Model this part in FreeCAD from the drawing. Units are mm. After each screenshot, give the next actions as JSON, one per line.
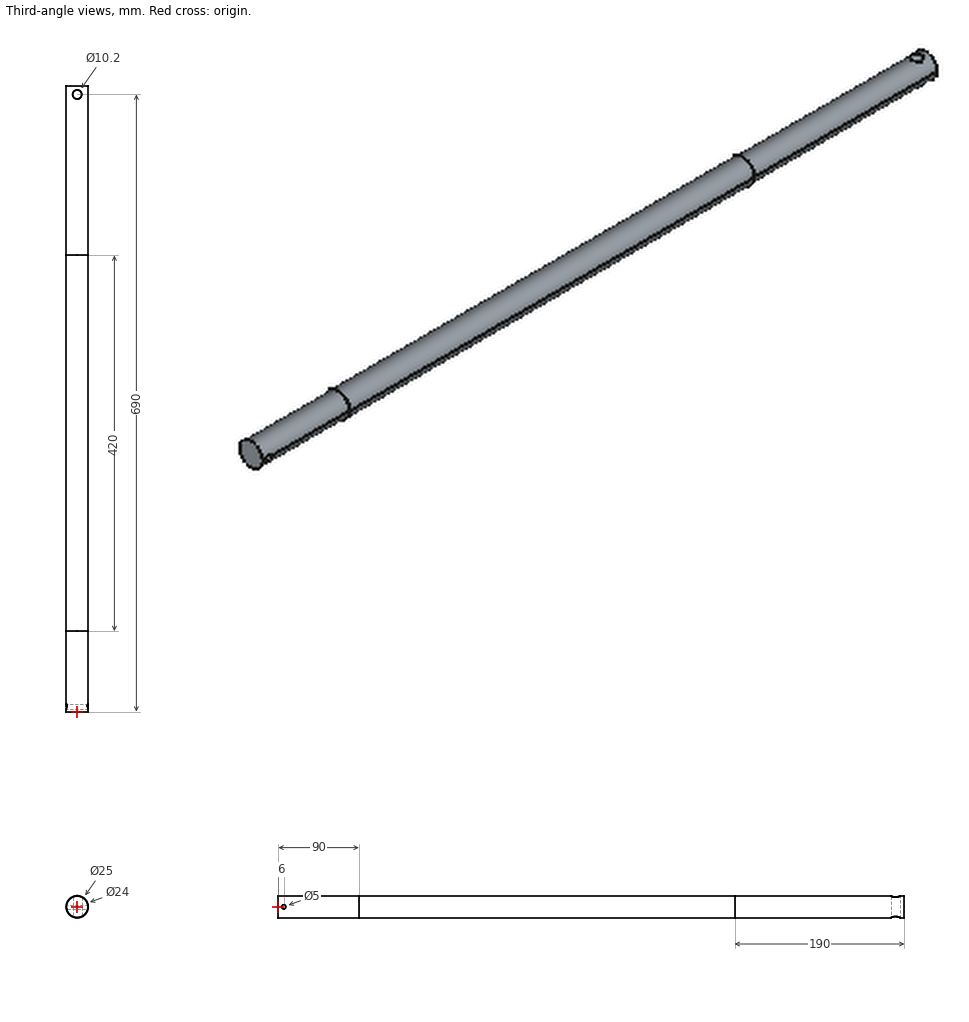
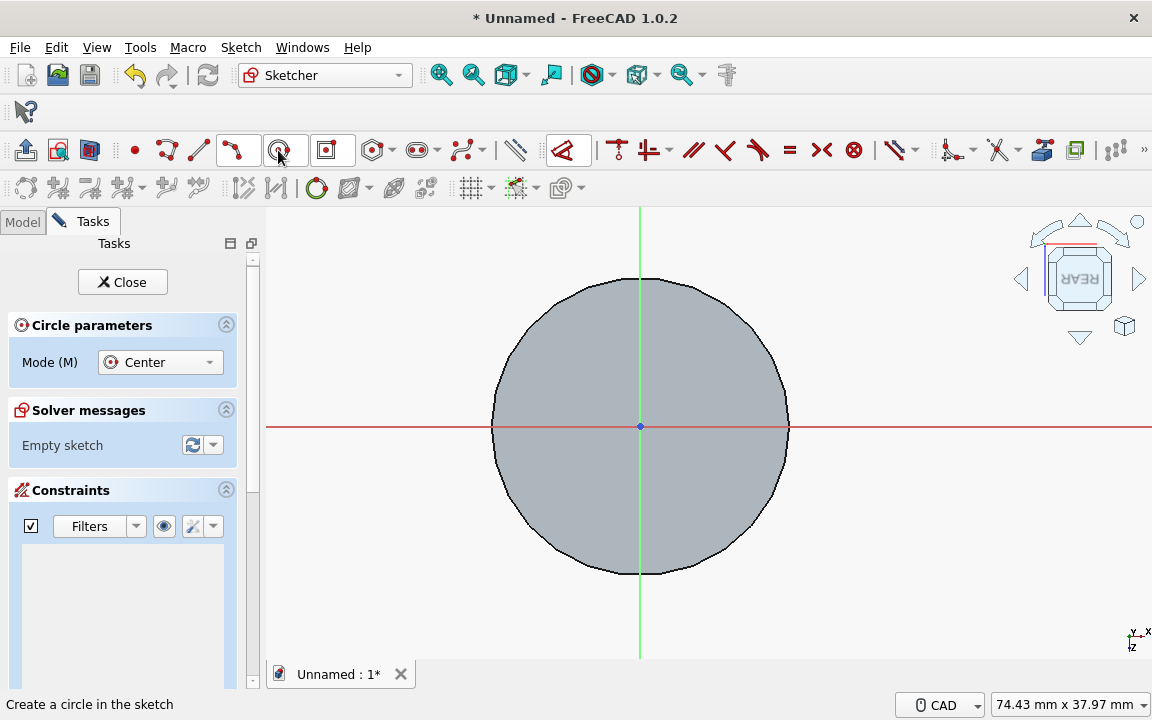
{"action": "left_click", "coordinate": [640, 427]}
{"action": "left_click", "coordinate": [741, 326]}
{"action": "key", "text": "Escape"}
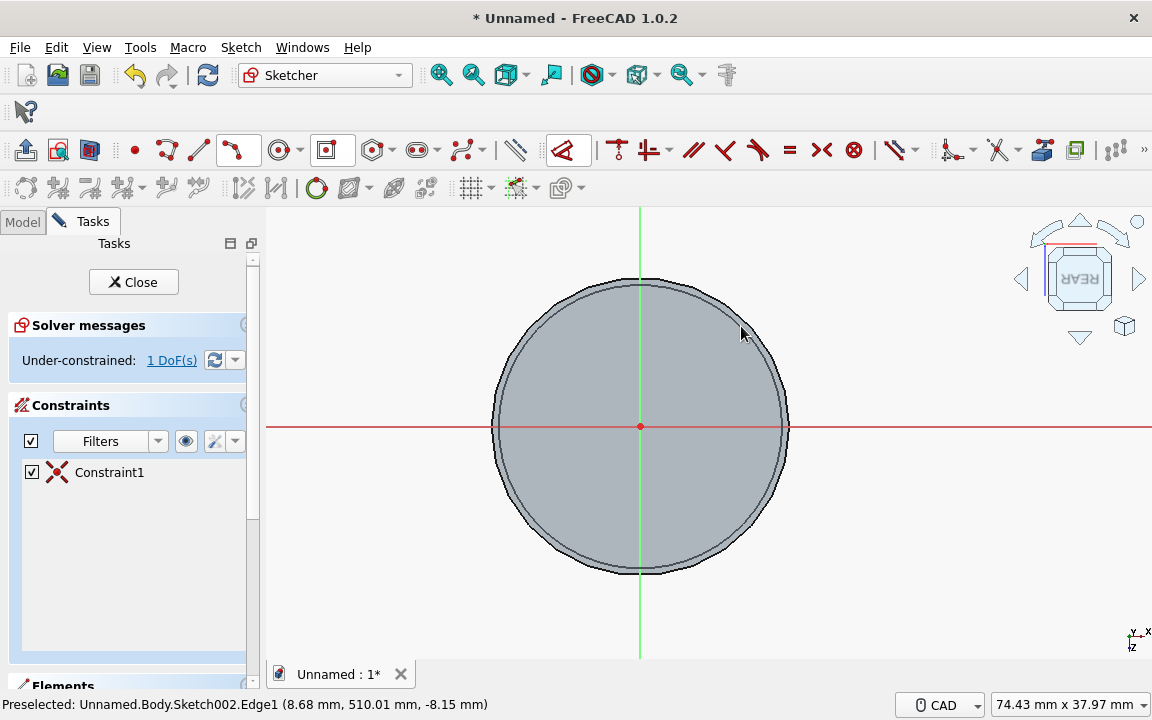
{"action": "left_click", "coordinate": [740, 326]}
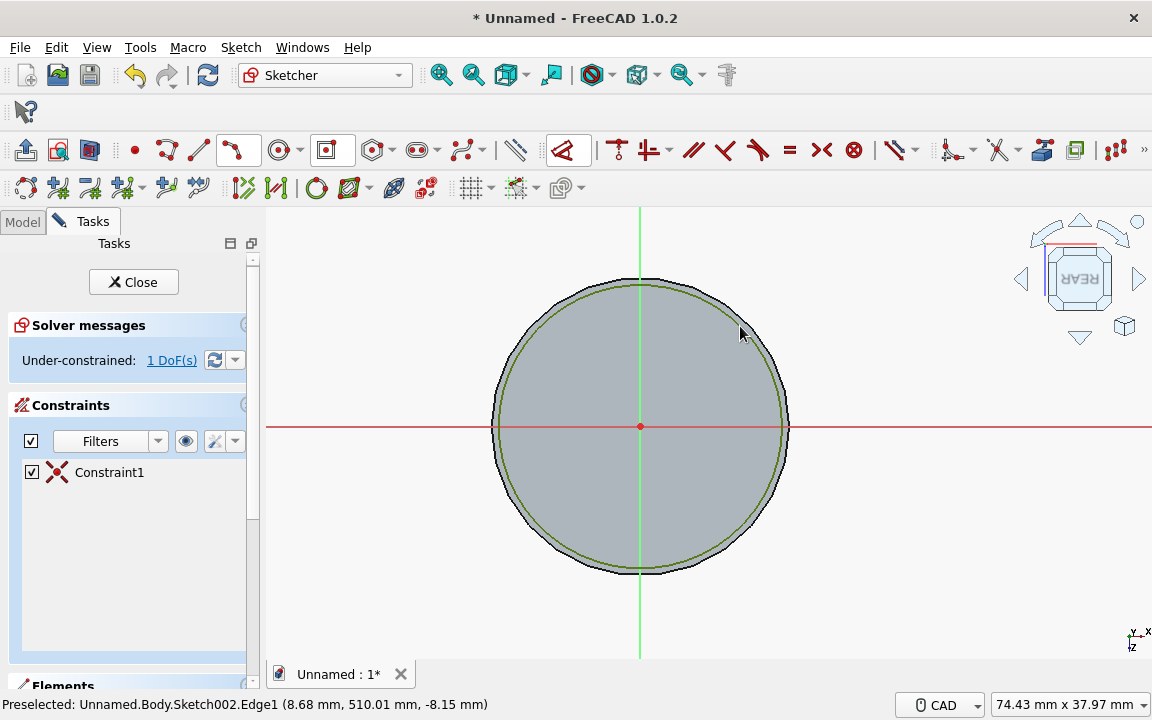
{"action": "key", "text": "k o"}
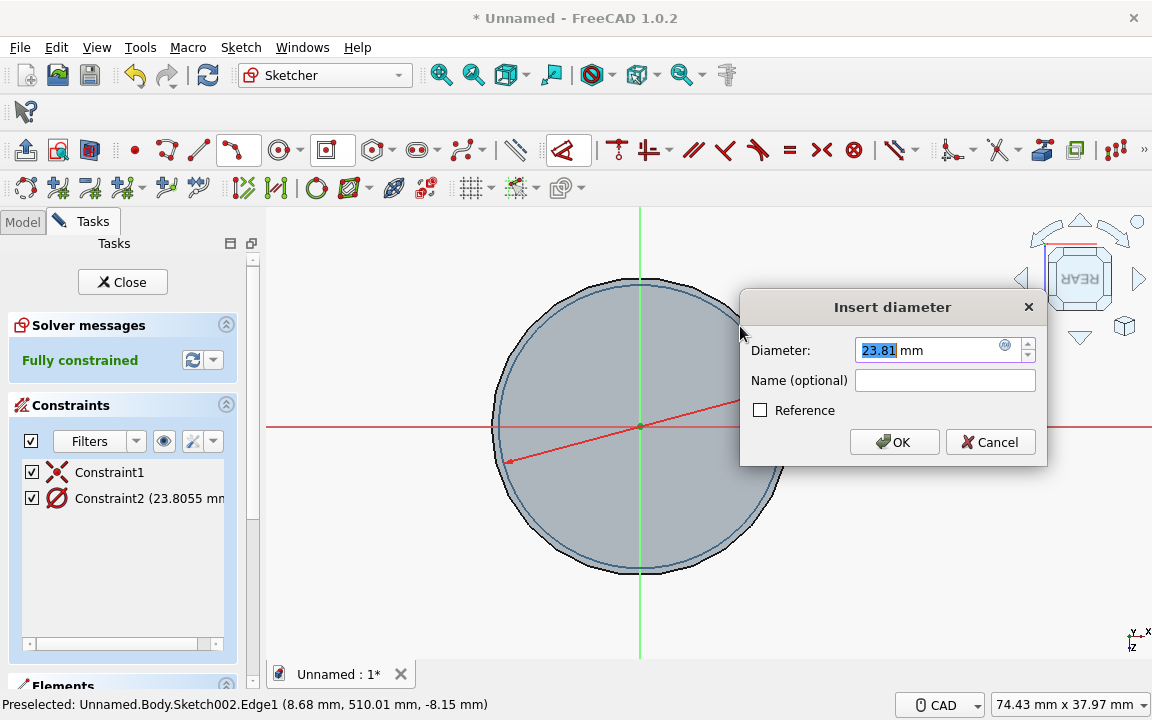
{"action": "type", "text": "24"}
{"action": "key", "text": "Return"}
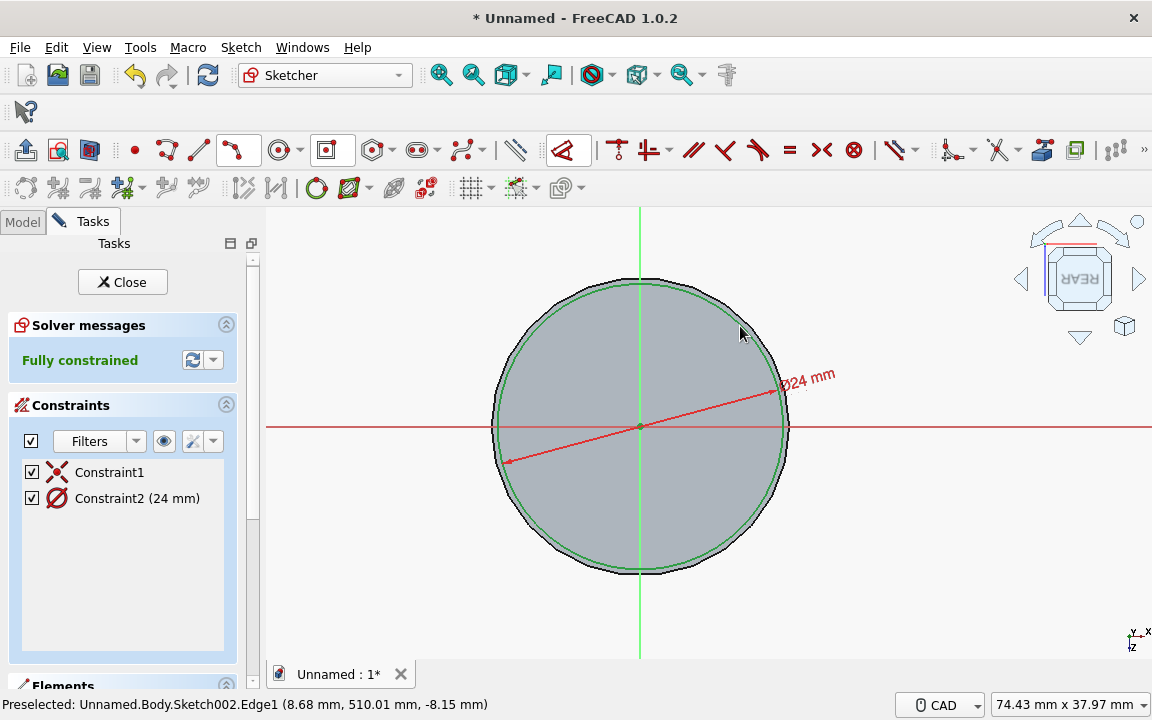
{"action": "left_click", "coordinate": [123, 282]}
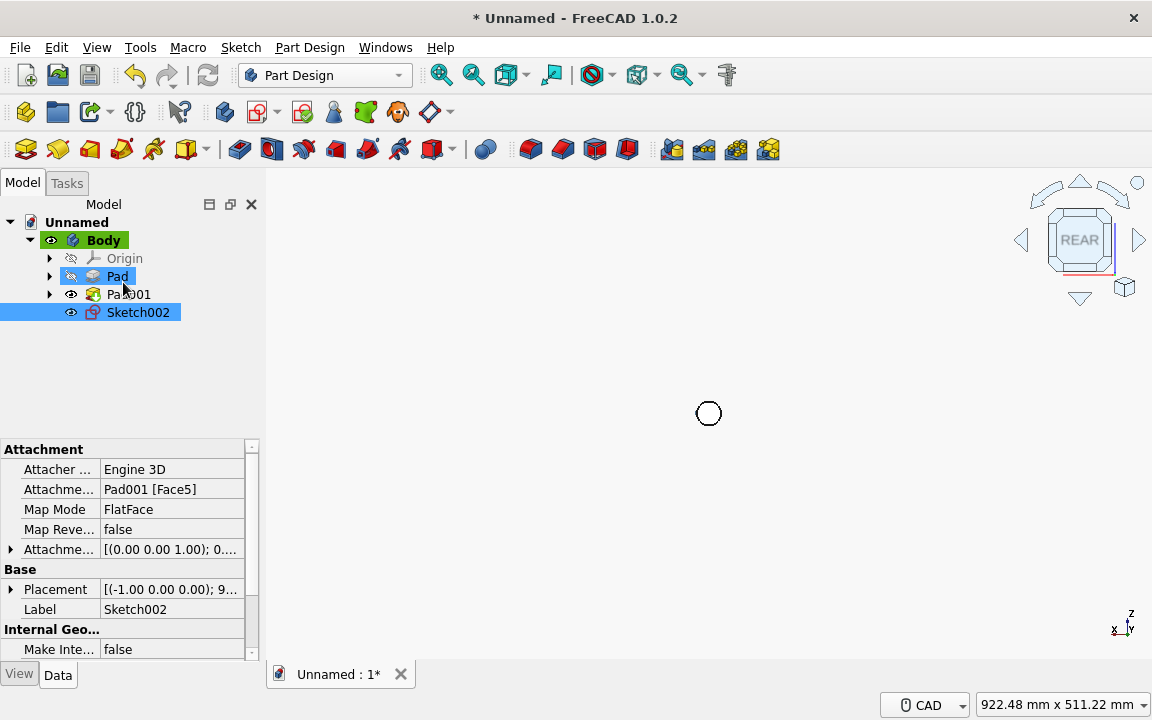
{"action": "left_click", "coordinate": [26, 150]}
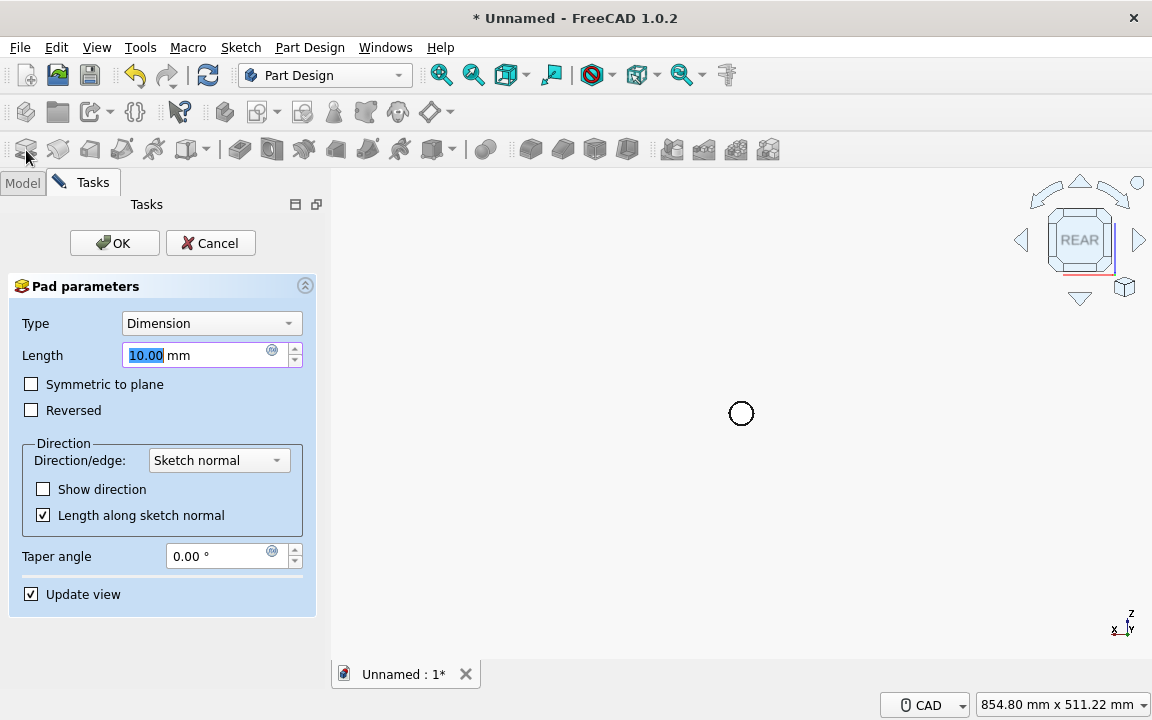
{"action": "type", "text": "190"}
{"action": "key", "text": "Tab"}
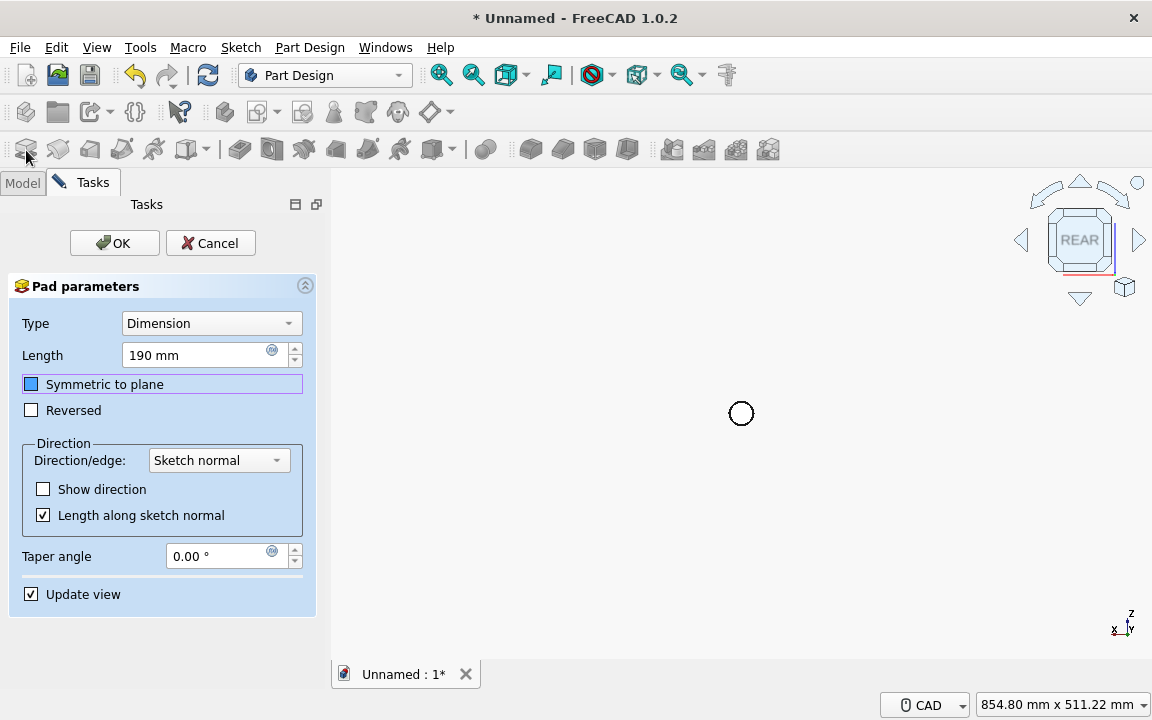
{"action": "left_click", "coordinate": [115, 243]}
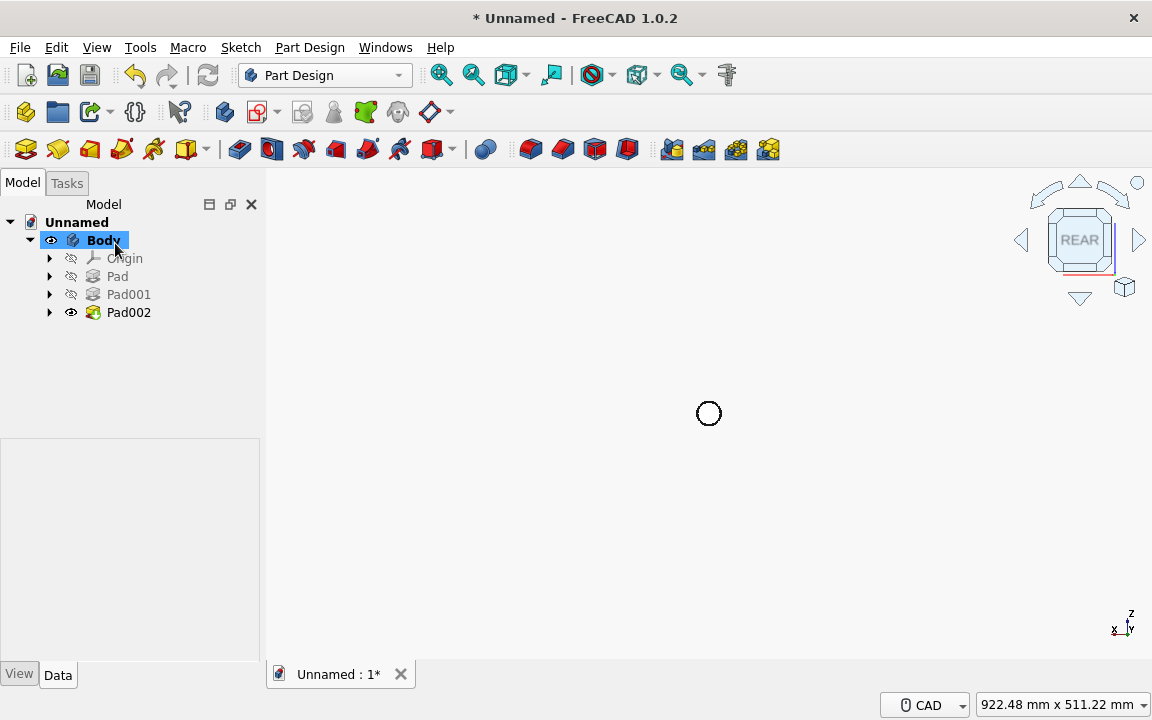
{"action": "left_click", "coordinate": [442, 76]}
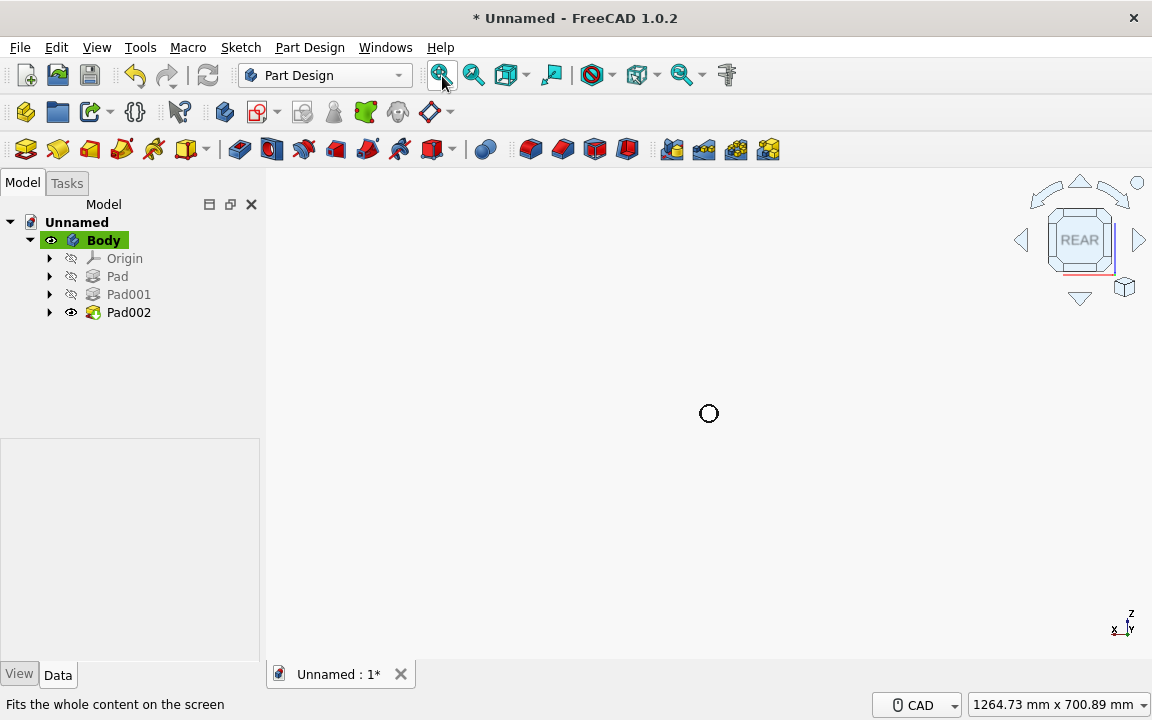
{"action": "left_click", "coordinate": [258, 112]}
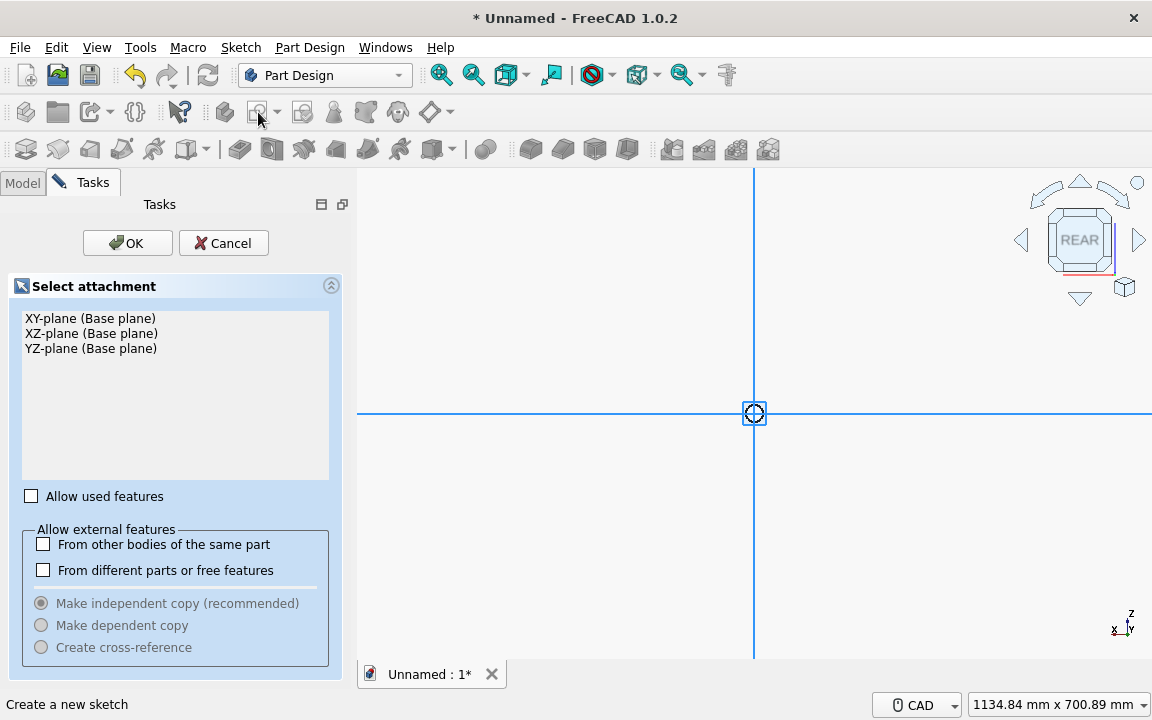
{"action": "left_click", "coordinate": [82, 318]}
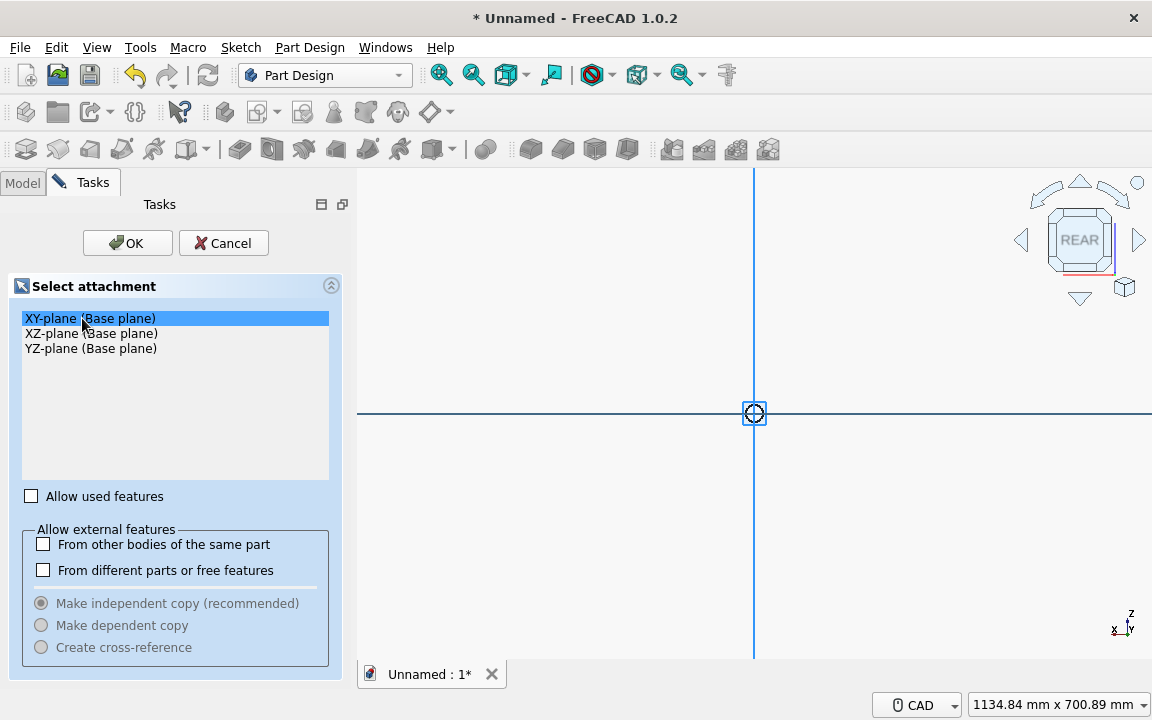
{"action": "left_click", "coordinate": [128, 243]}